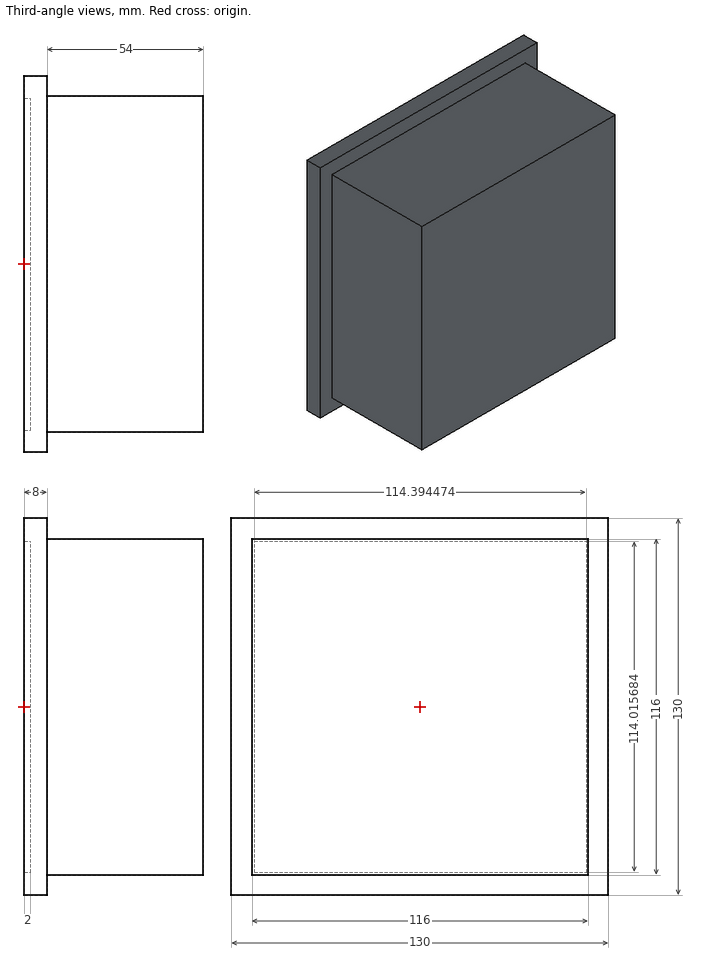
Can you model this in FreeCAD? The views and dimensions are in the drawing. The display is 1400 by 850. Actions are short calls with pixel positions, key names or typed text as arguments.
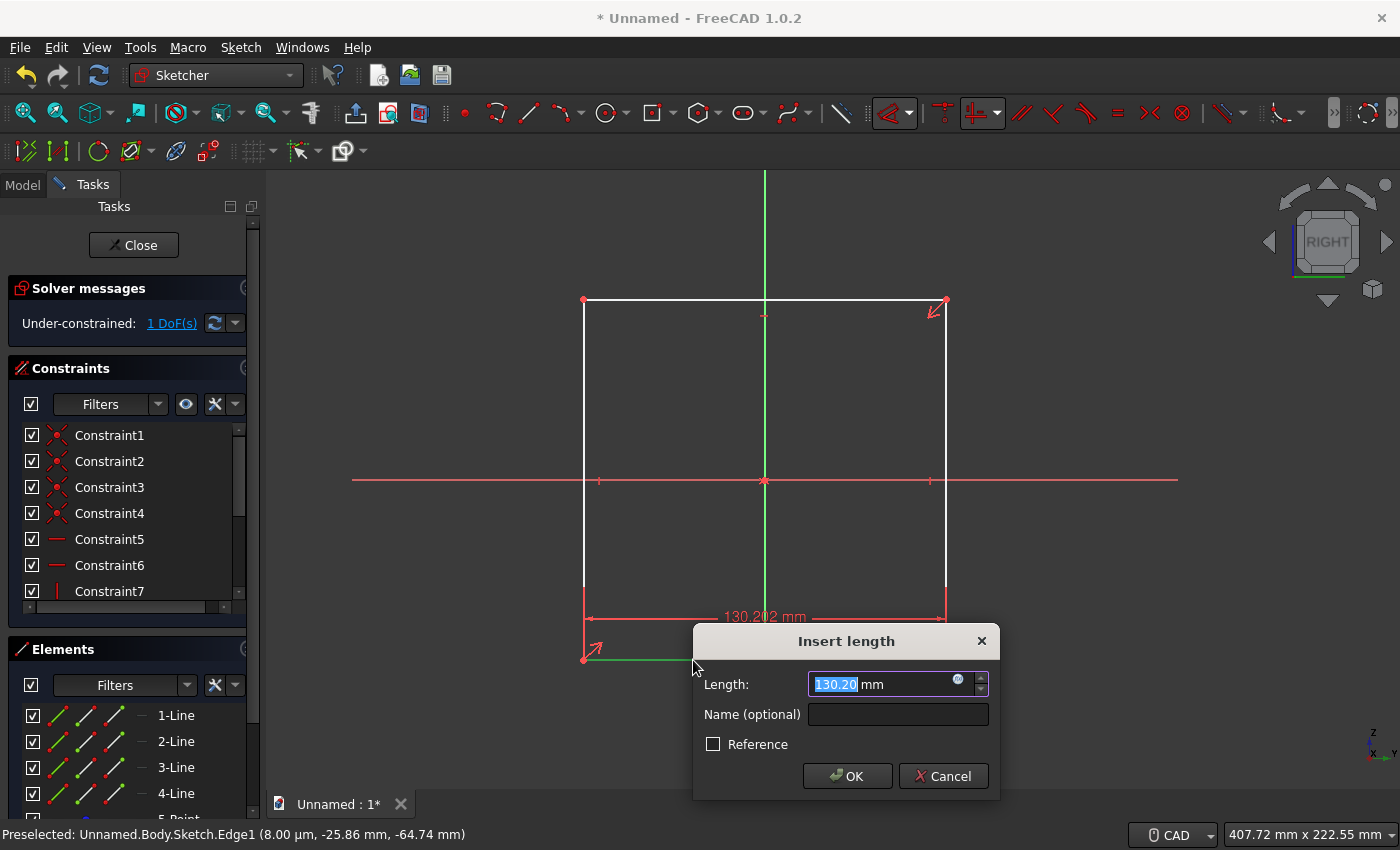
text(130)
key(Return)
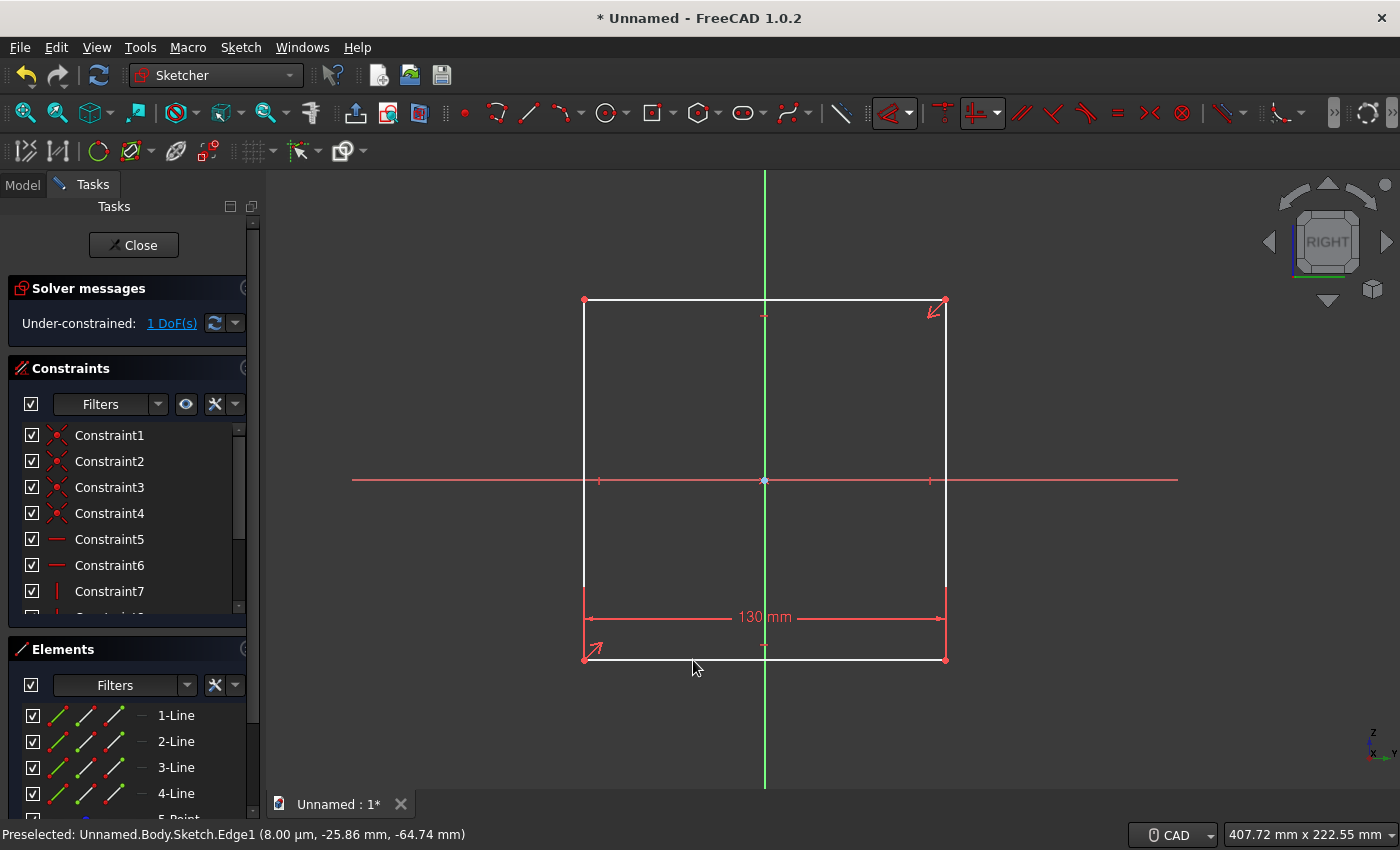
click(946, 552)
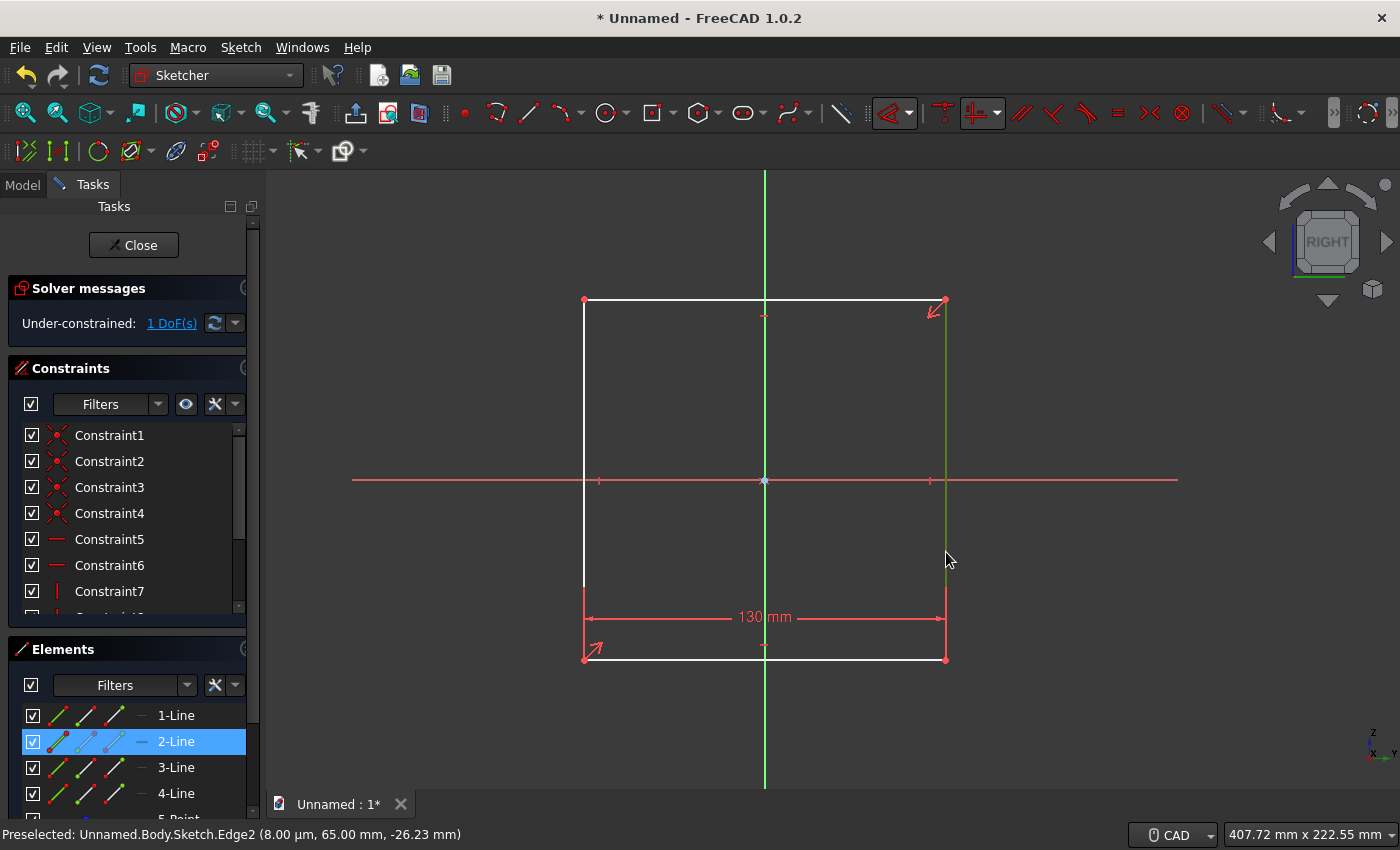
key(i)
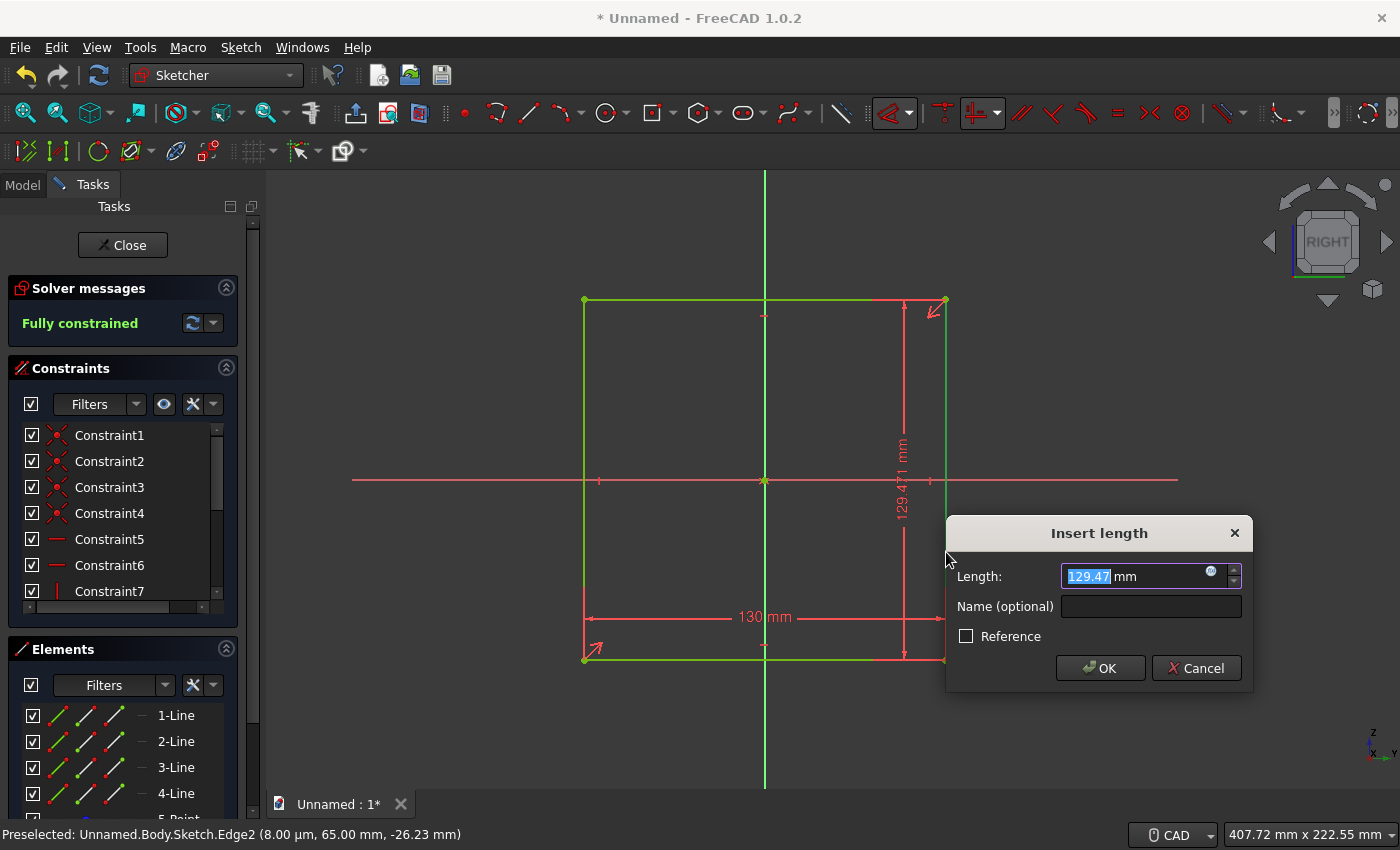
text(130)
key(Return)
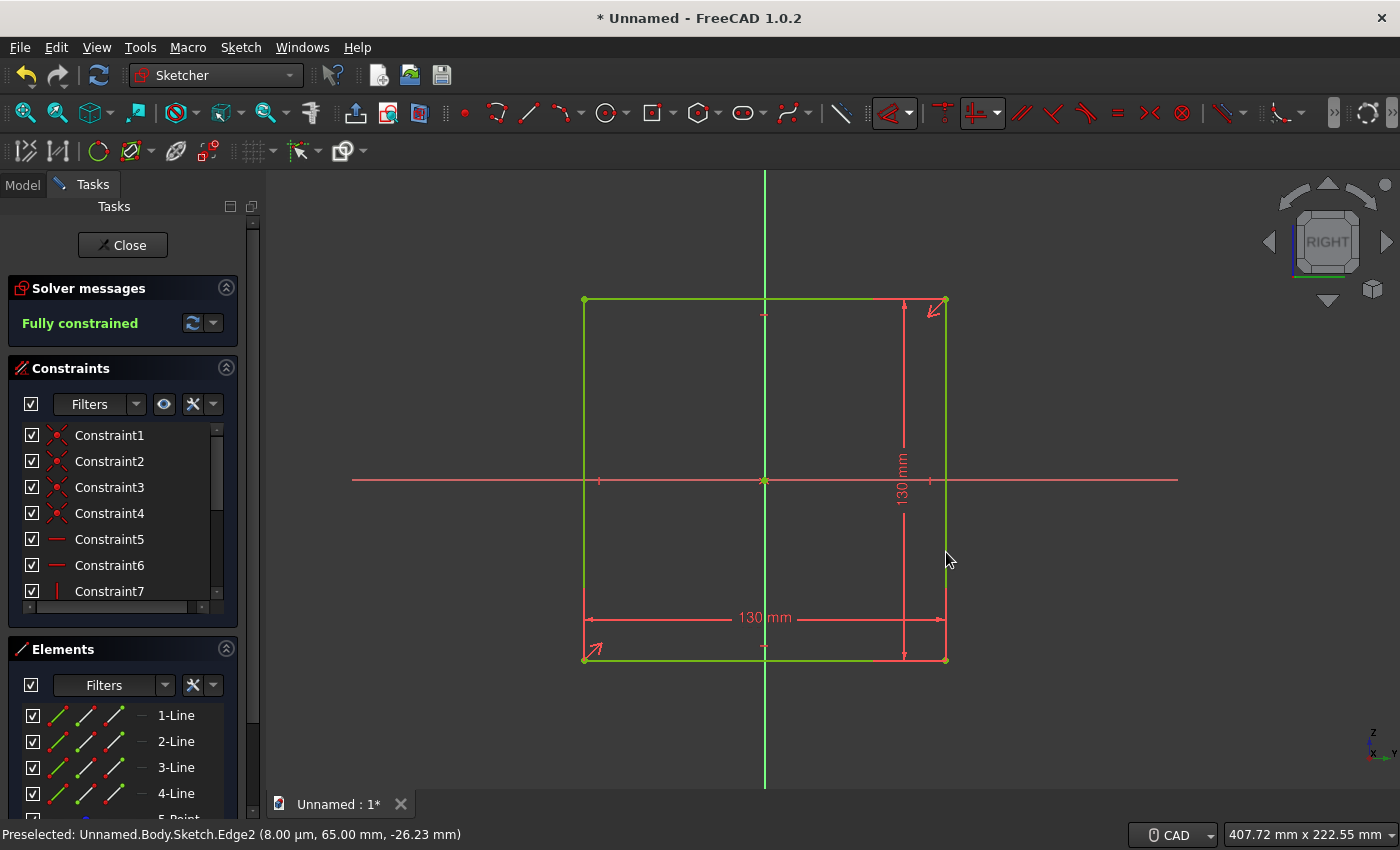
click(123, 245)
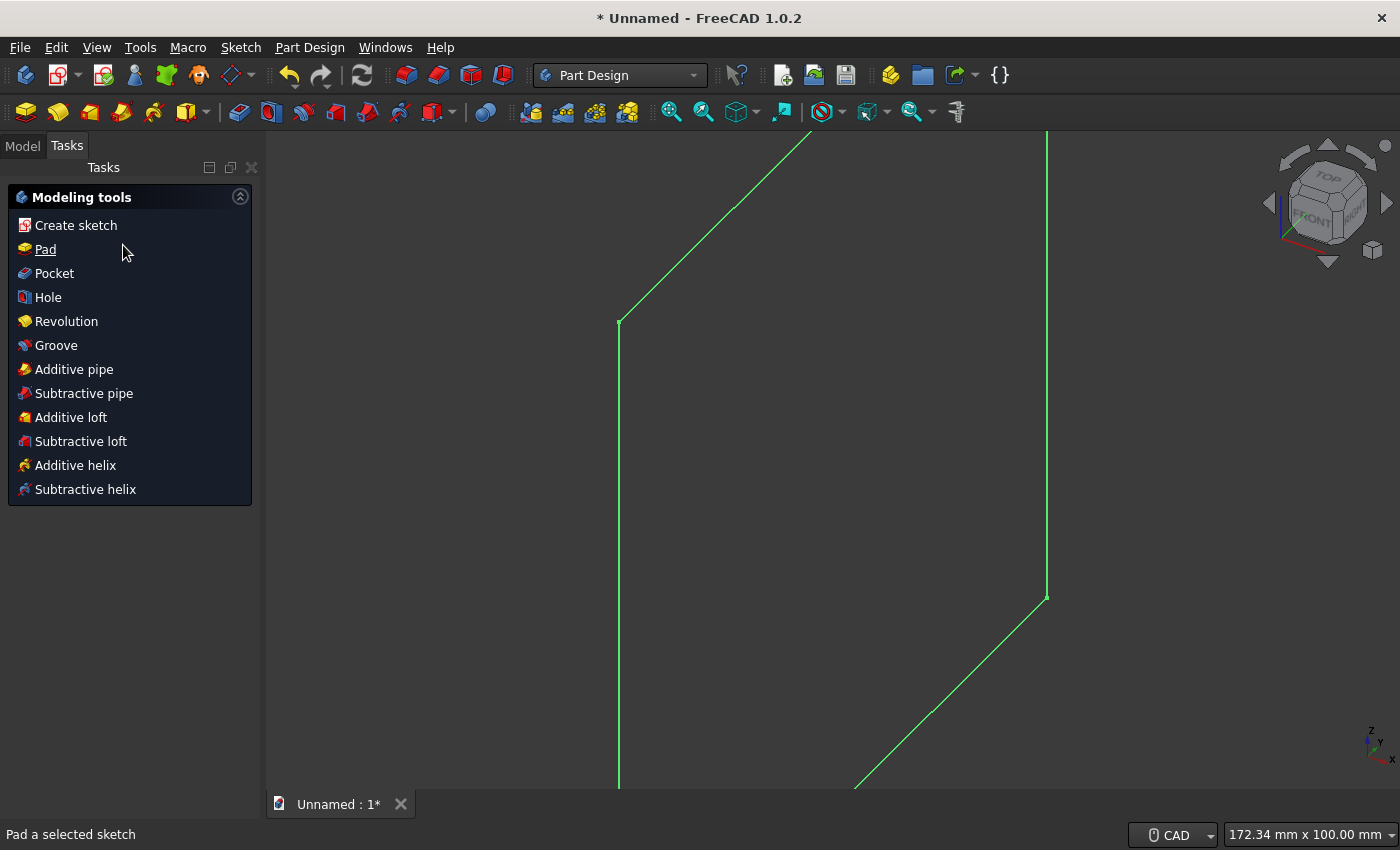
click(26, 112)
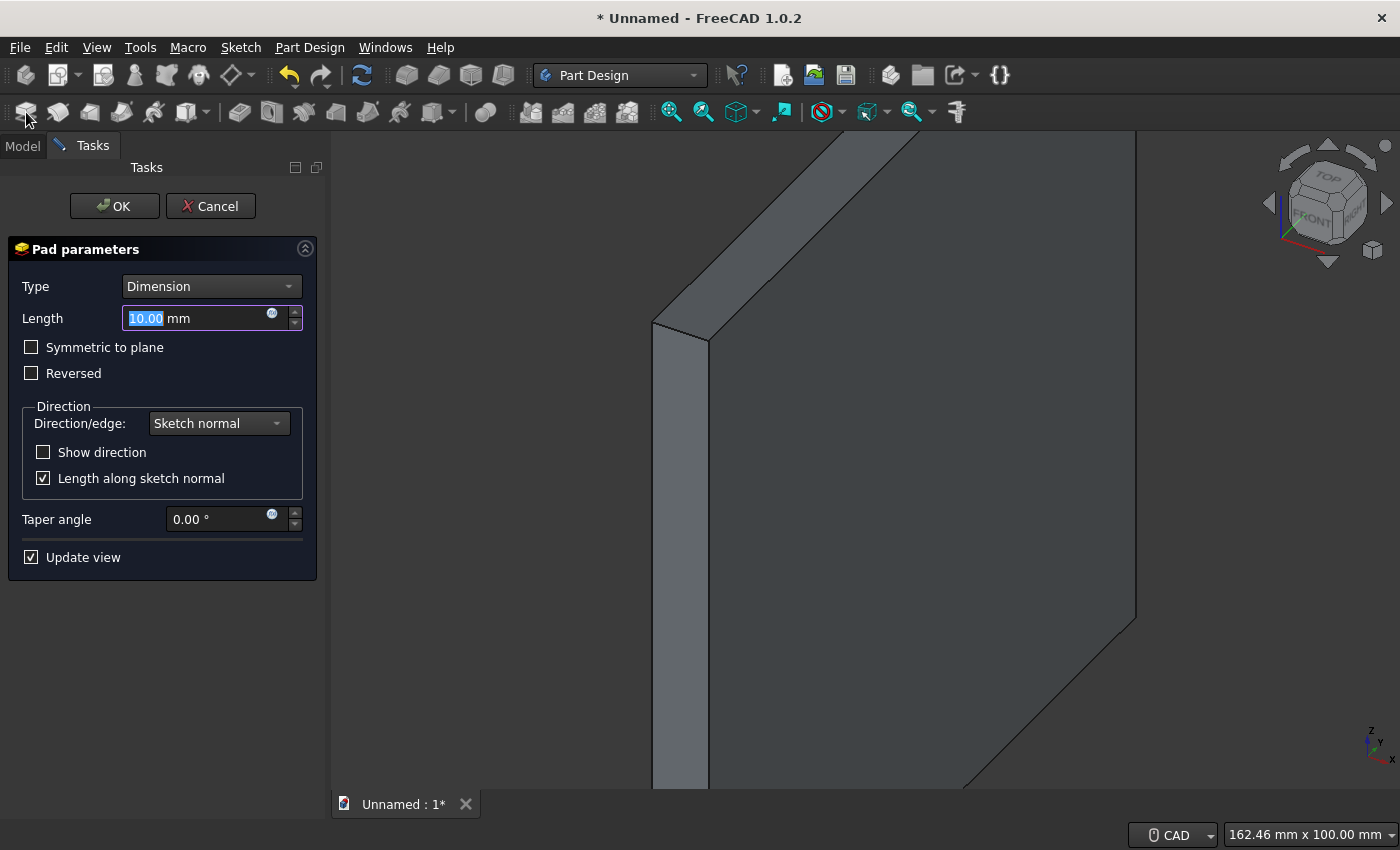
text(8)
key(Tab)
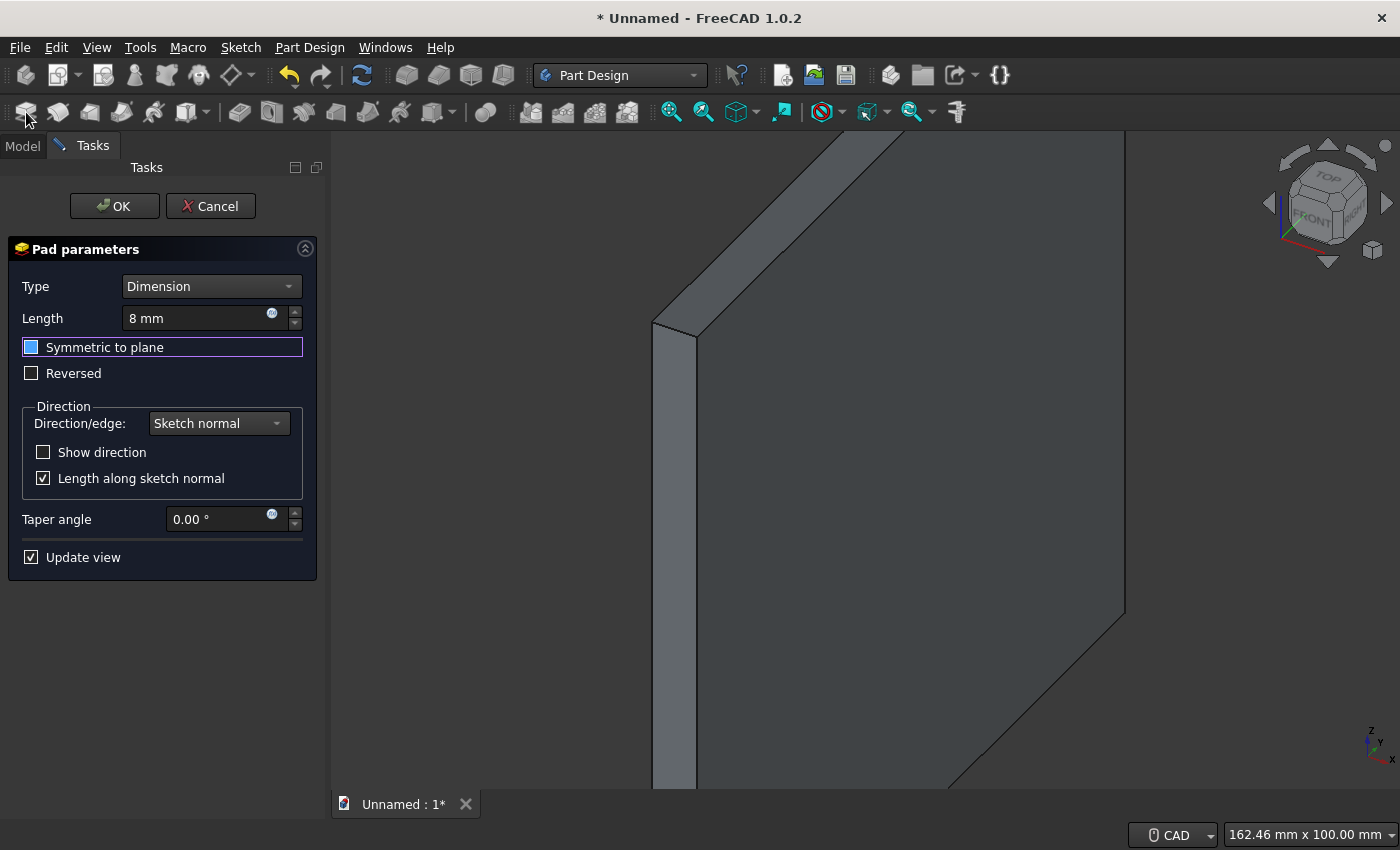
click(115, 206)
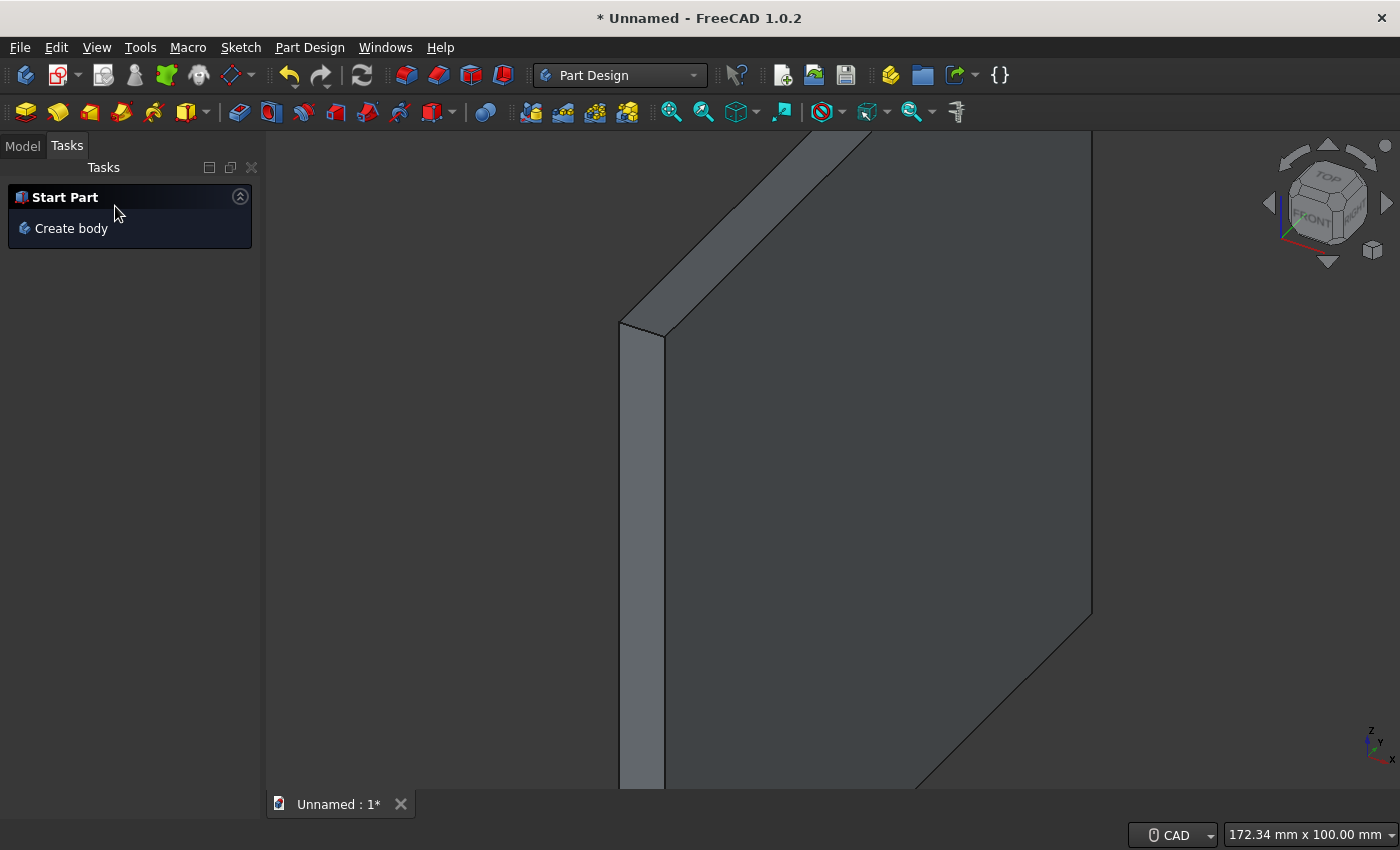
click(672, 112)